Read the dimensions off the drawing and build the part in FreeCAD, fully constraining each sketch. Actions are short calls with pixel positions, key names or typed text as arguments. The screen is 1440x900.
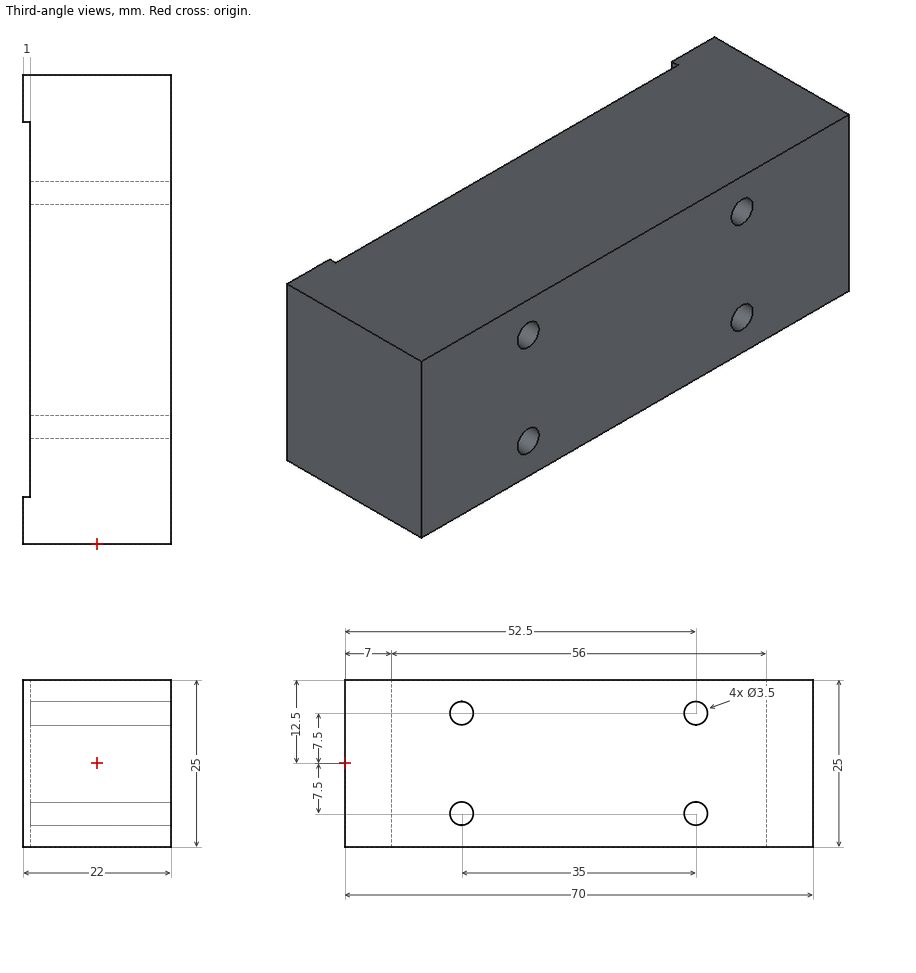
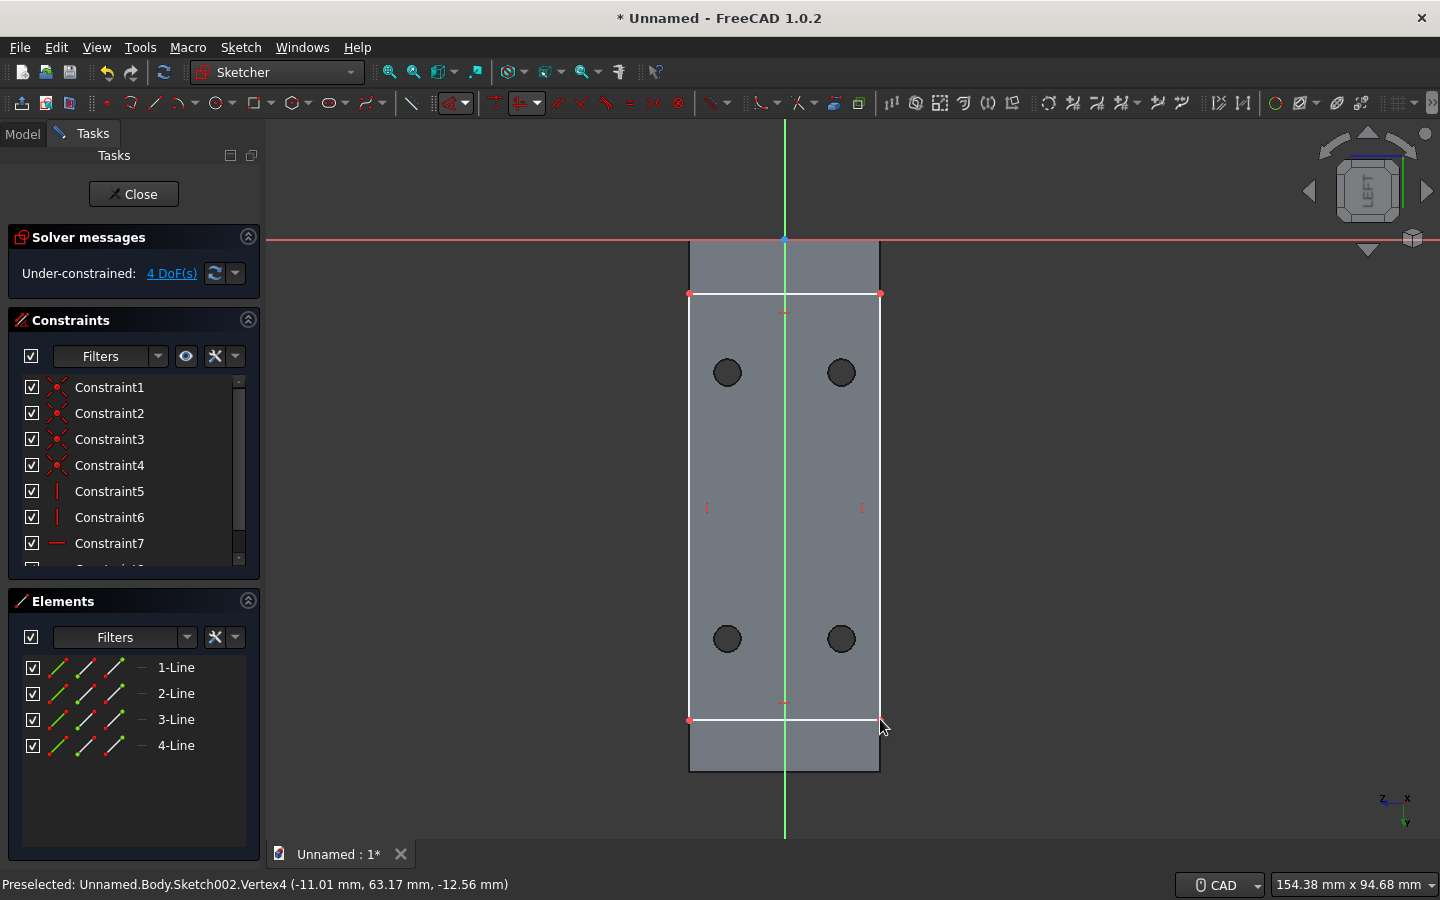
click(689, 422)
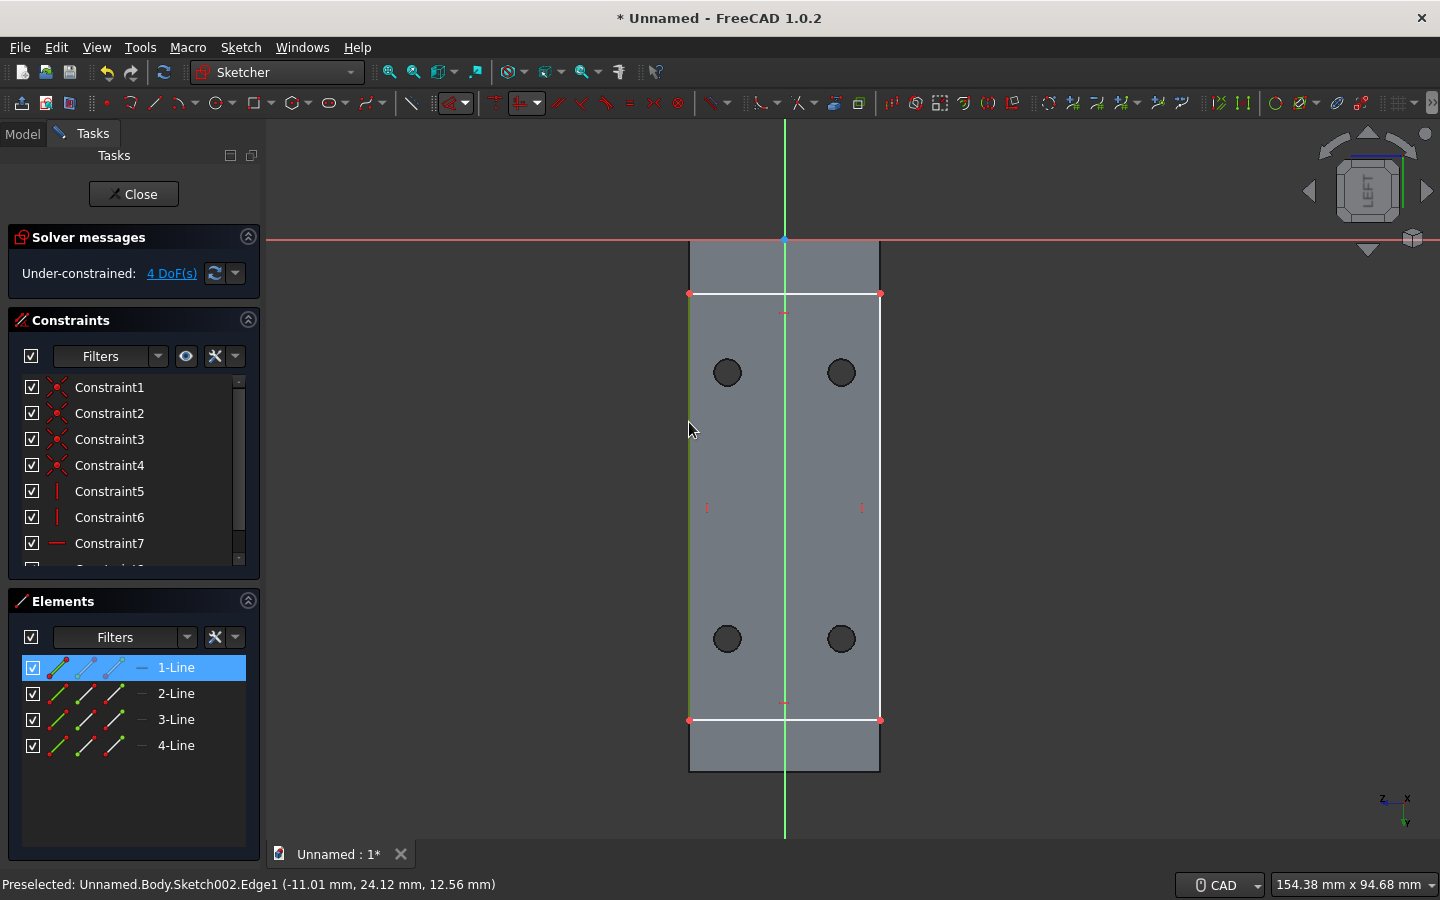
click(468, 104)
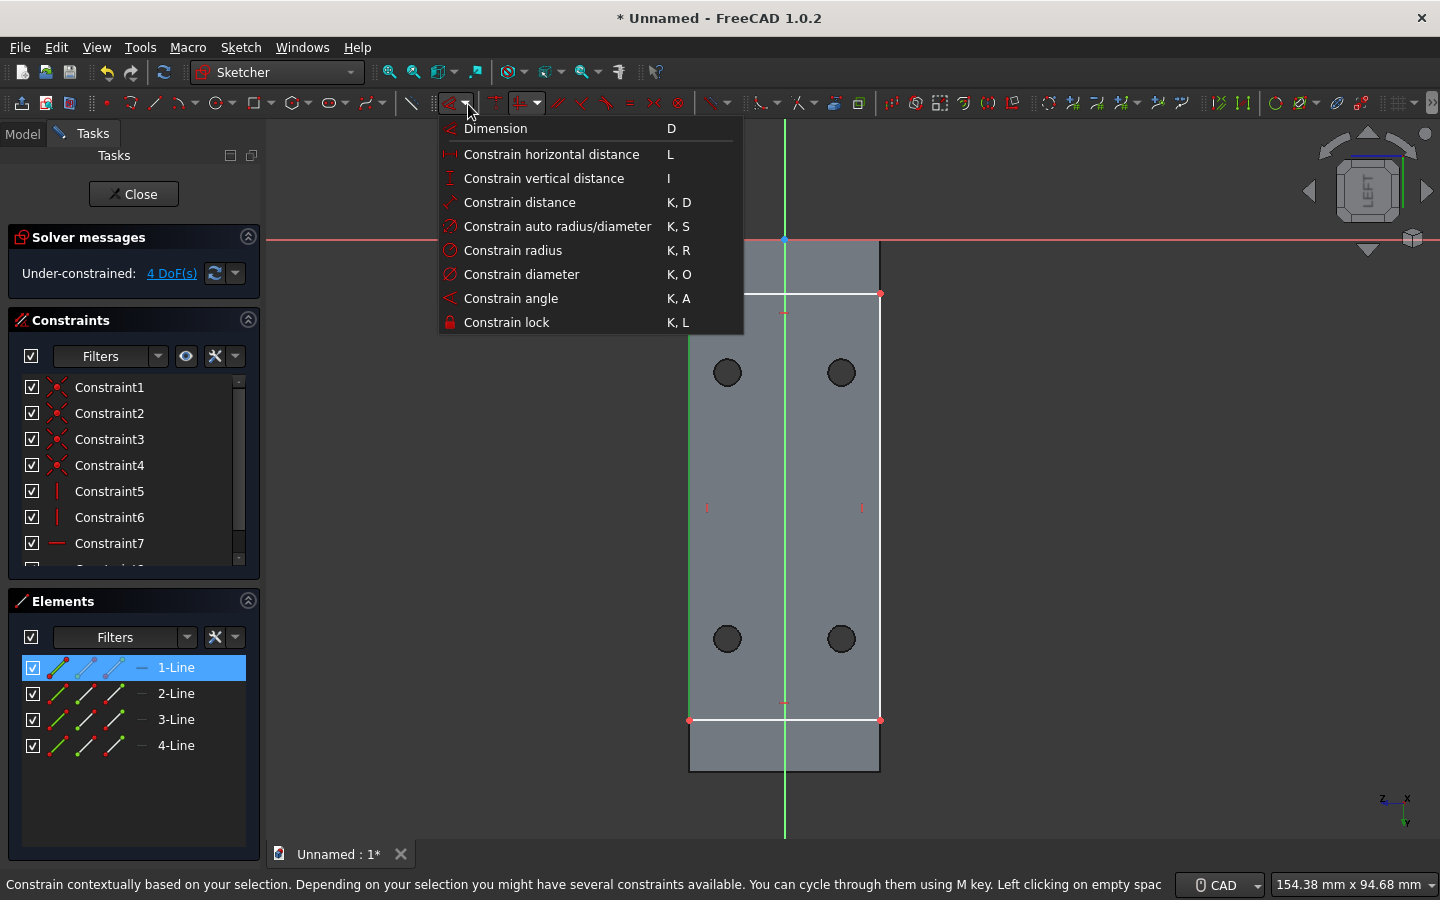
click(591, 178)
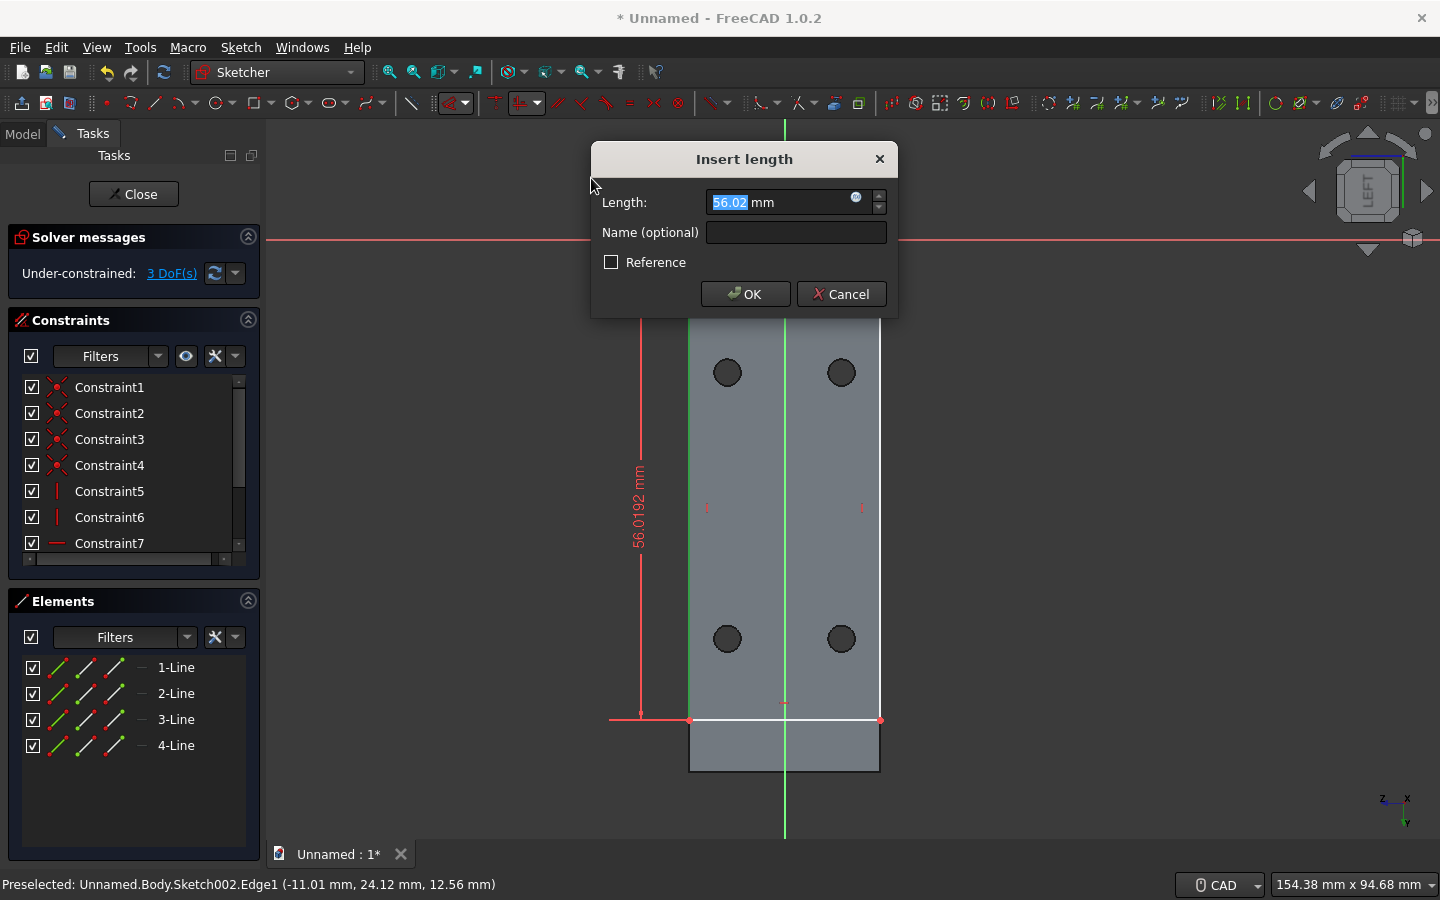
text(56)
key(Return)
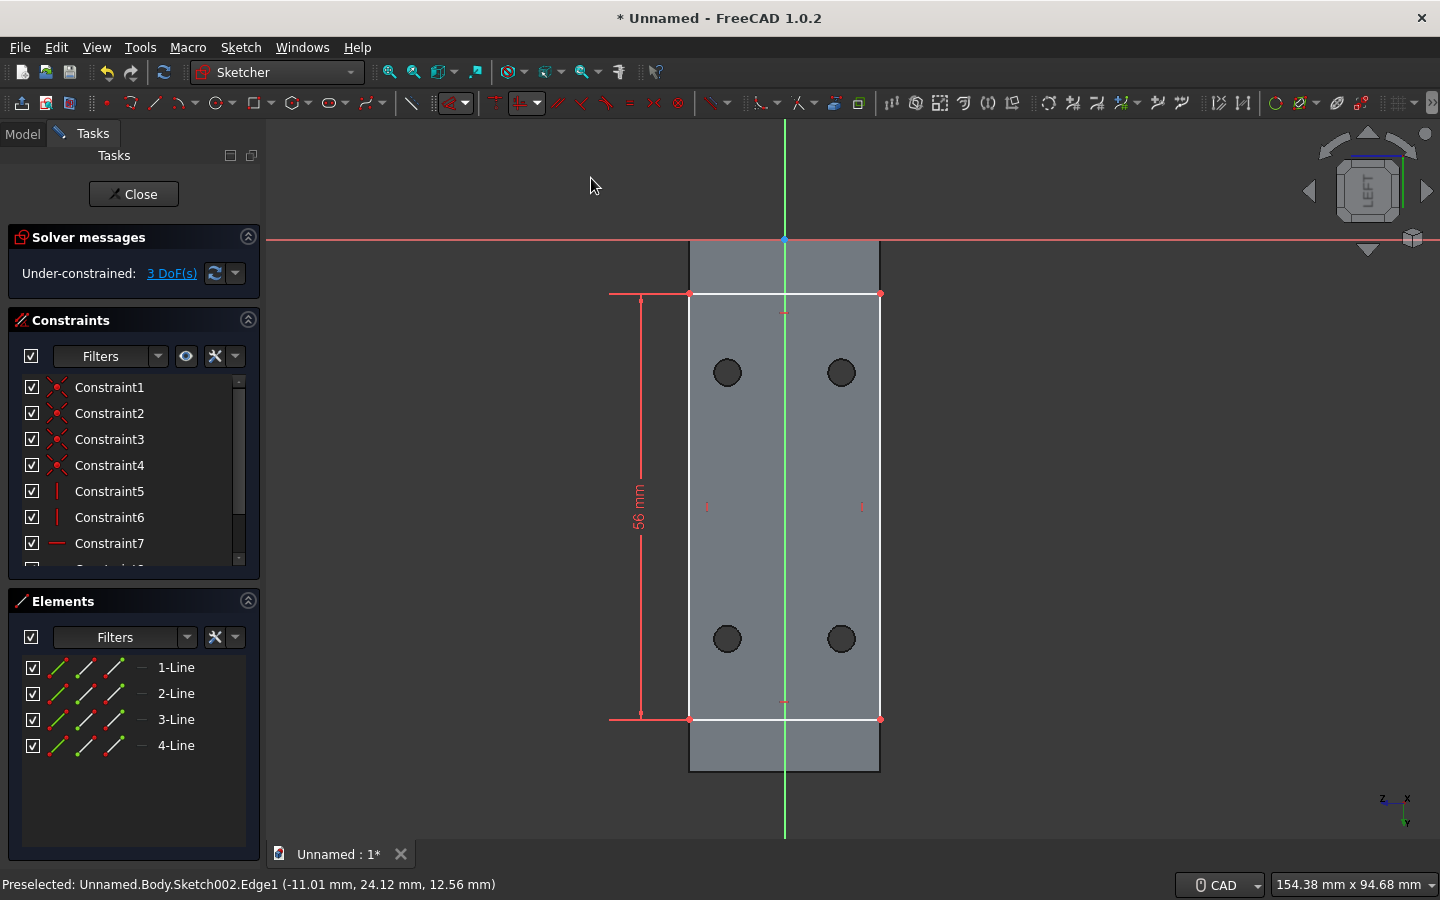
click(746, 720)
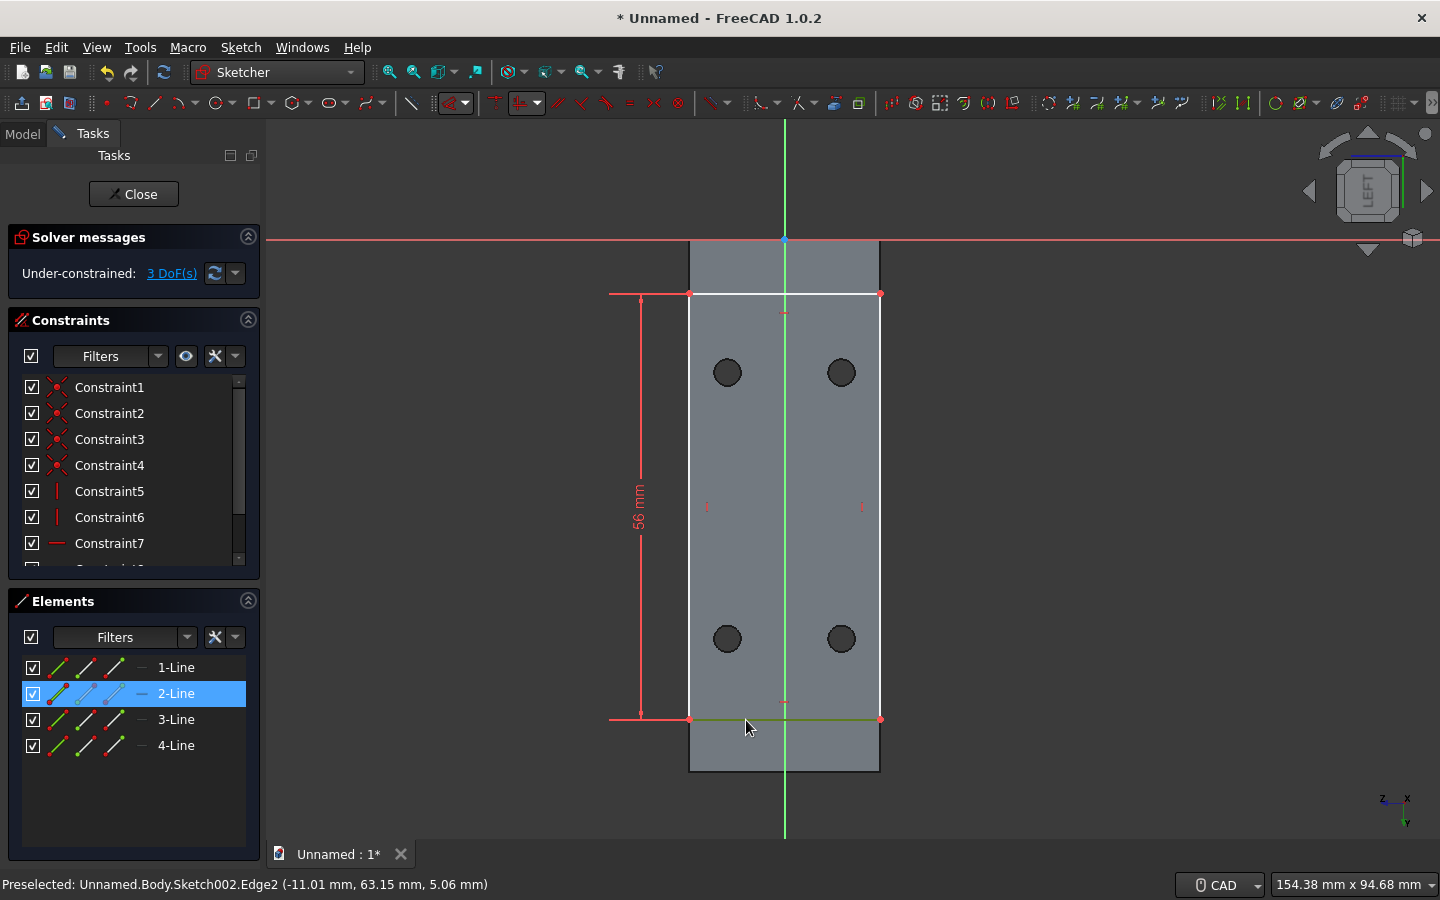
key(l)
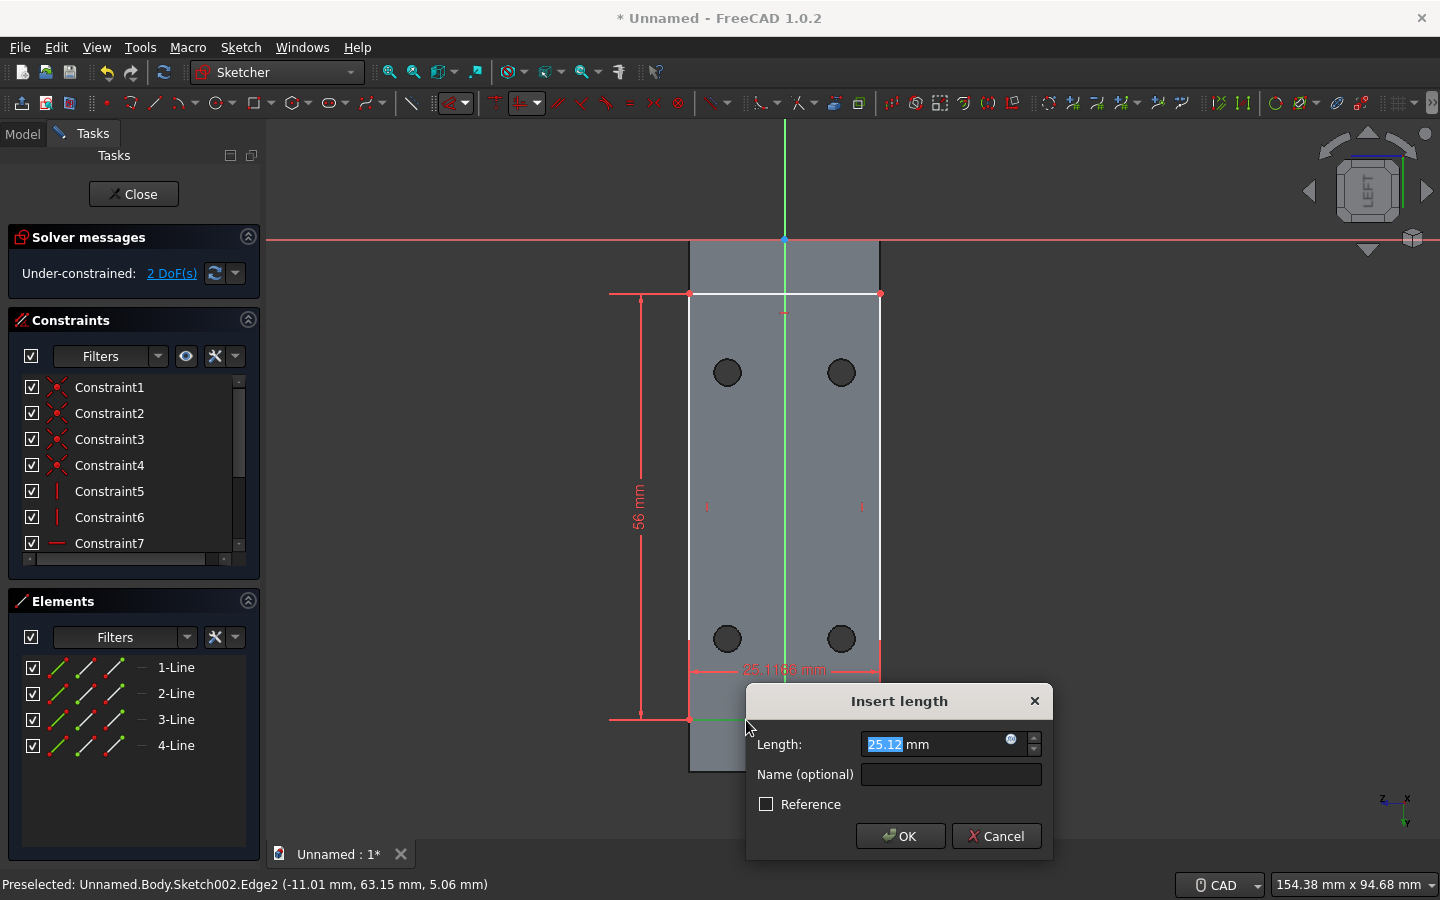
text(25)
key(Return)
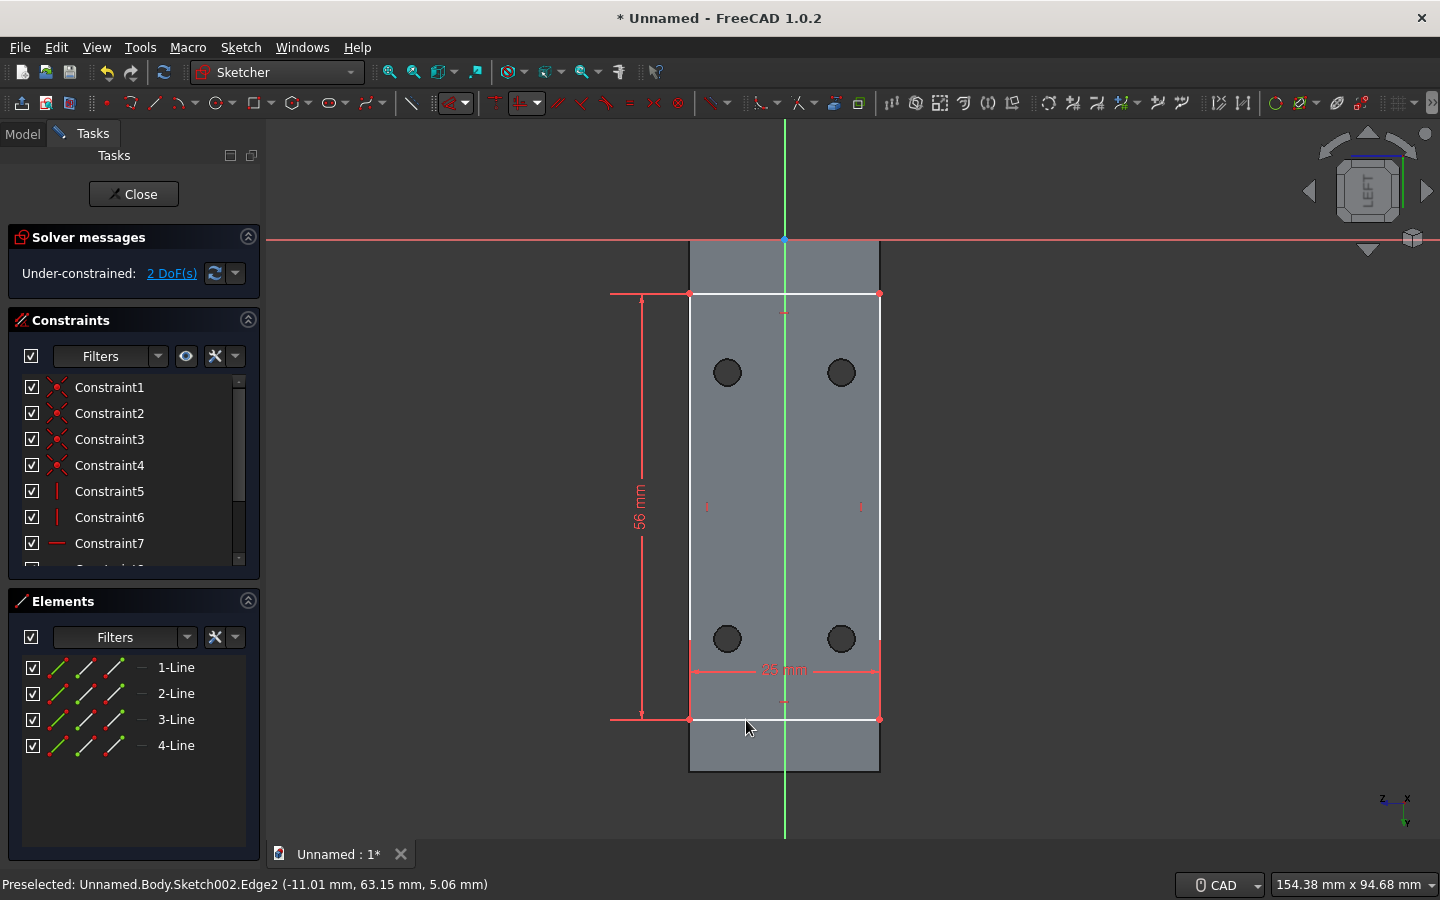
click(690, 294)